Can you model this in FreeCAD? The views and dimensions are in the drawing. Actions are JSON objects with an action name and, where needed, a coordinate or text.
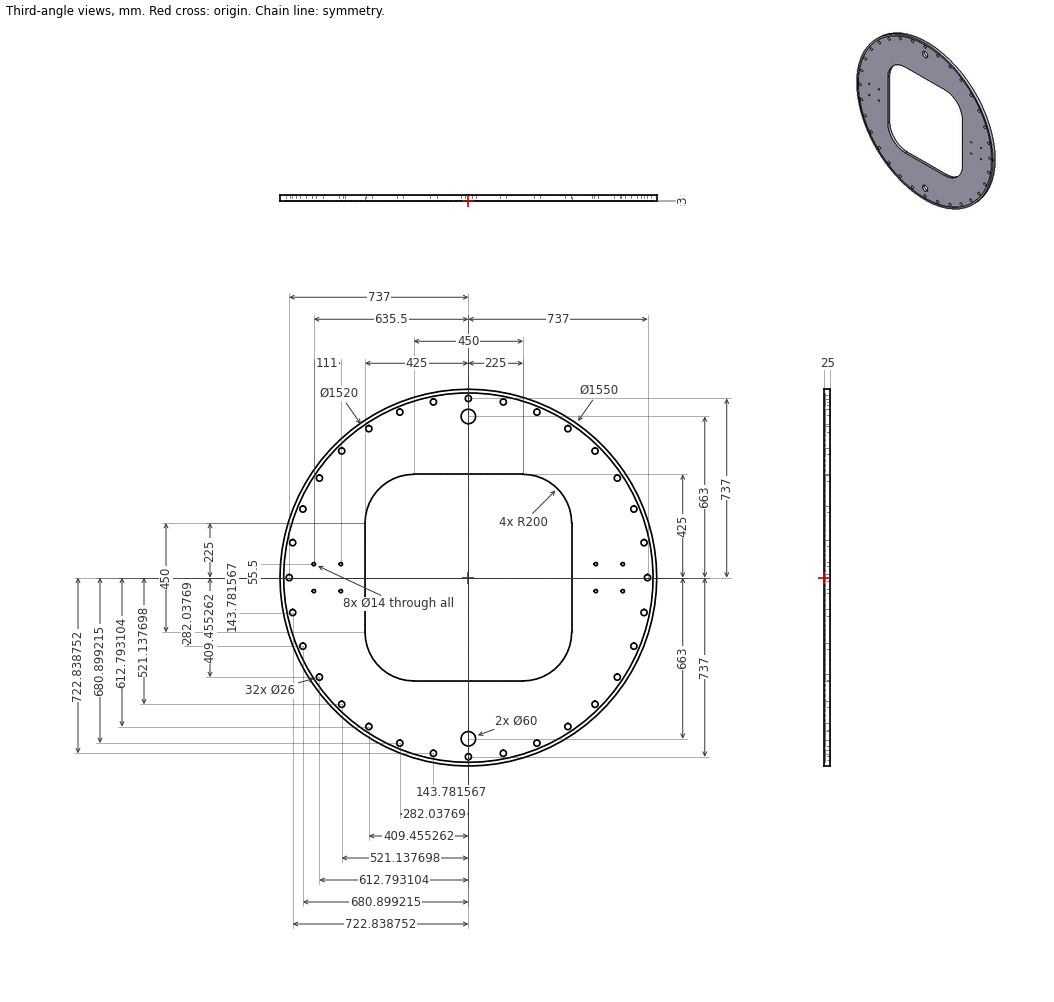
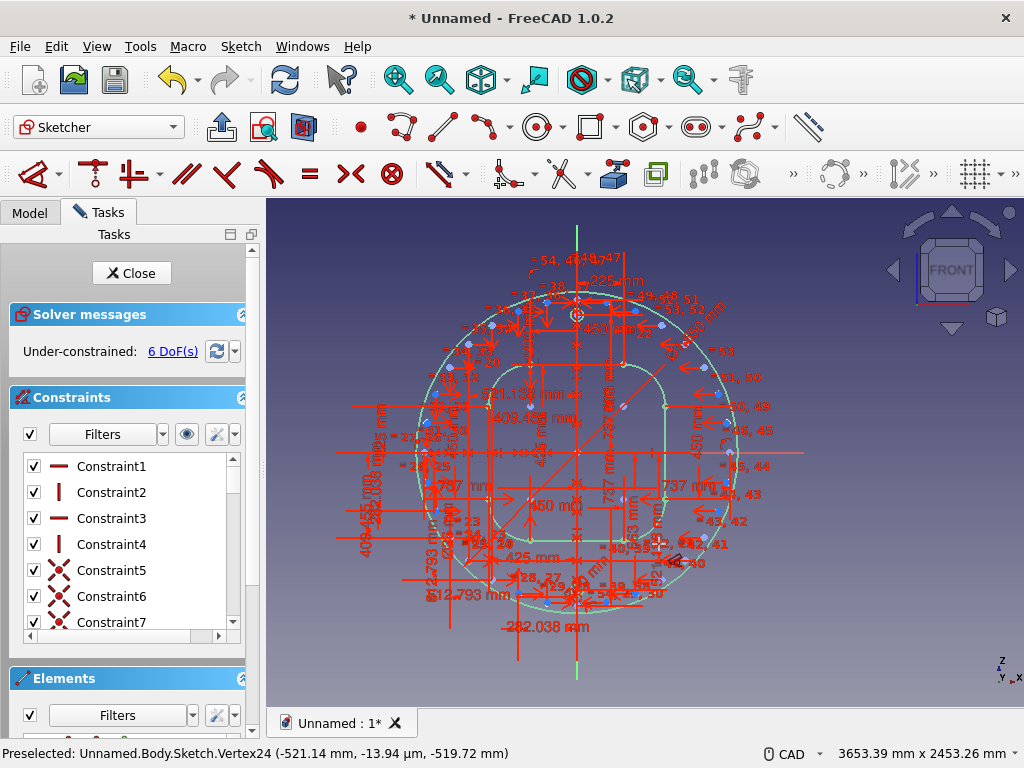
{"action": "left_click", "coordinate": [436, 511]}
{"action": "left_click", "coordinate": [474, 371]}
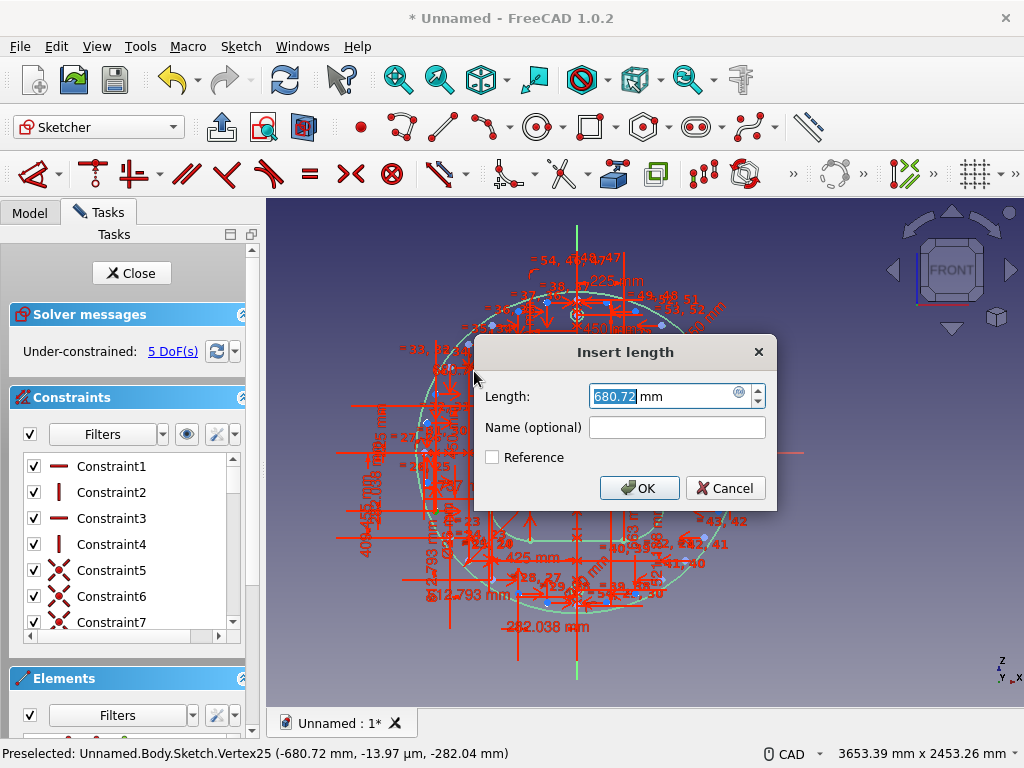
{"action": "type", "text": "680.899215"}
{"action": "key", "text": "Return"}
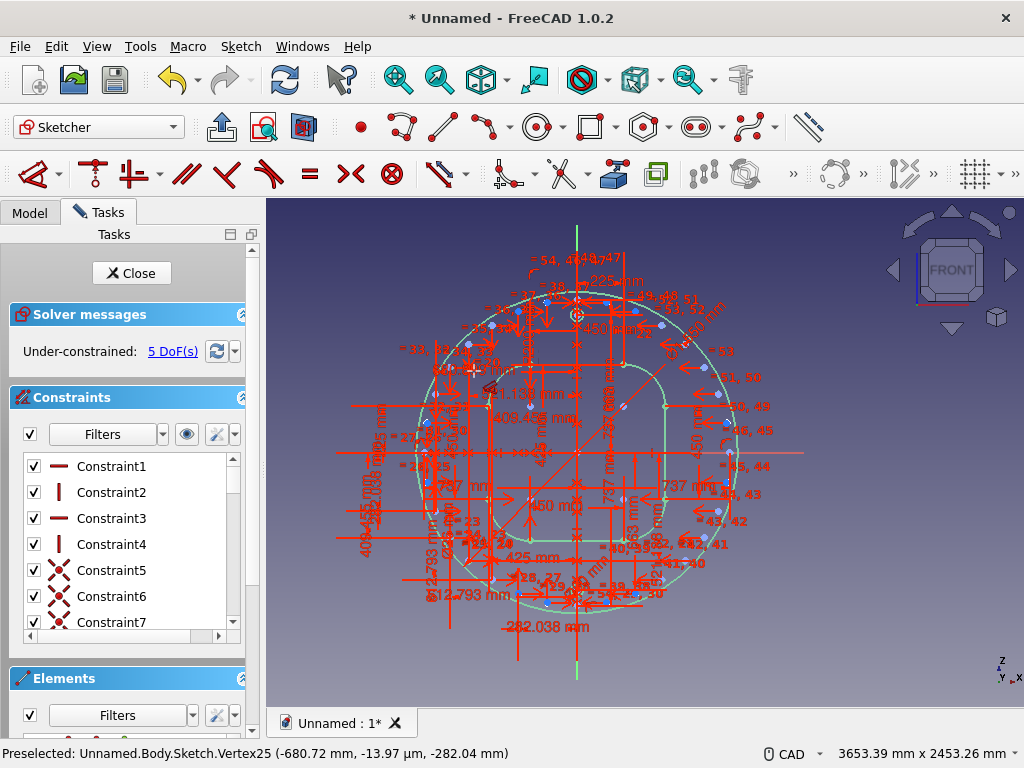
{"action": "left_click", "coordinate": [427, 483]}
{"action": "left_click", "coordinate": [450, 323]}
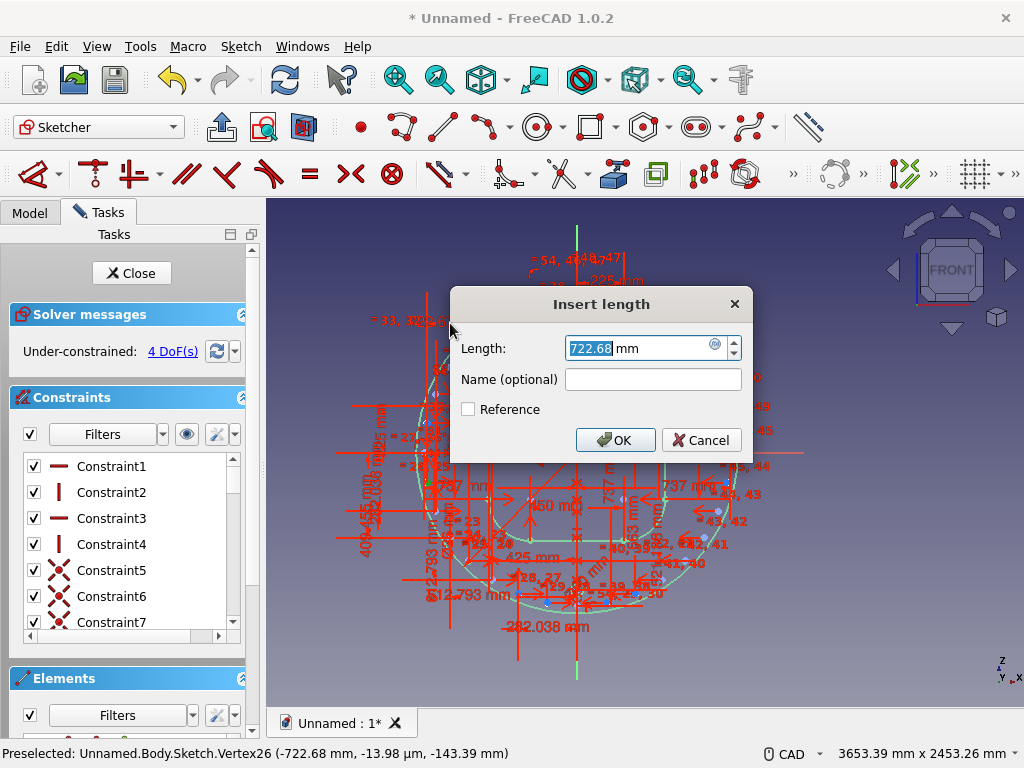
{"action": "type", "text": "722.838752"}
{"action": "key", "text": "Return"}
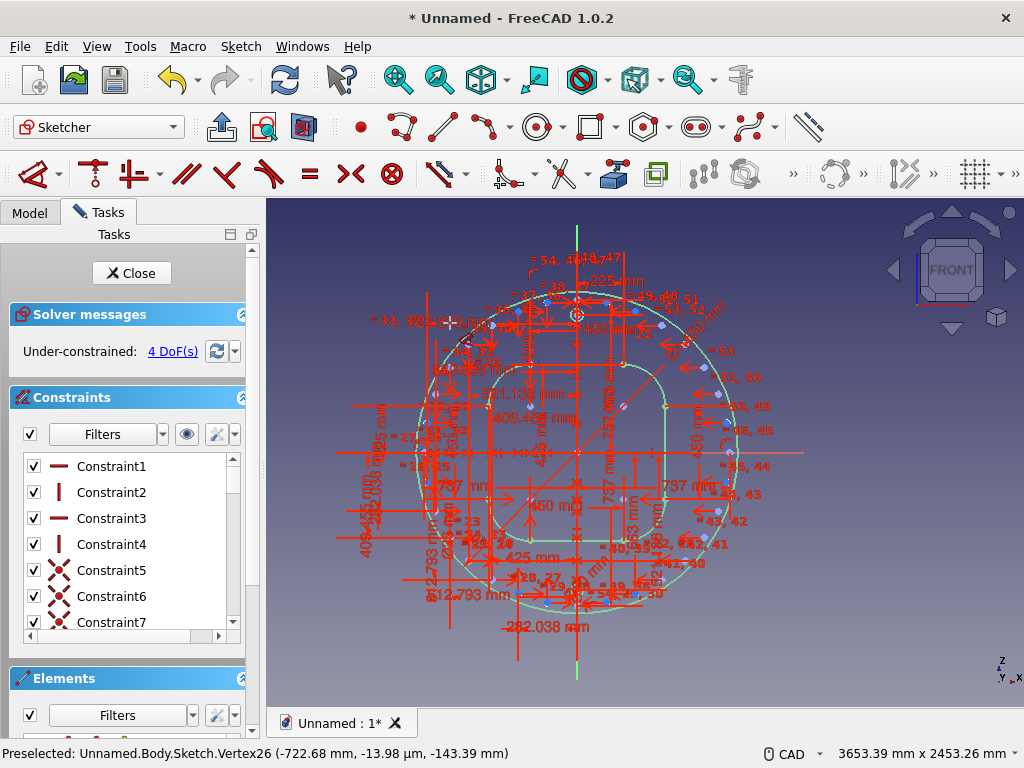
{"action": "scroll", "coordinate": [427, 483], "scroll_direction": "up", "scroll_amount": 2}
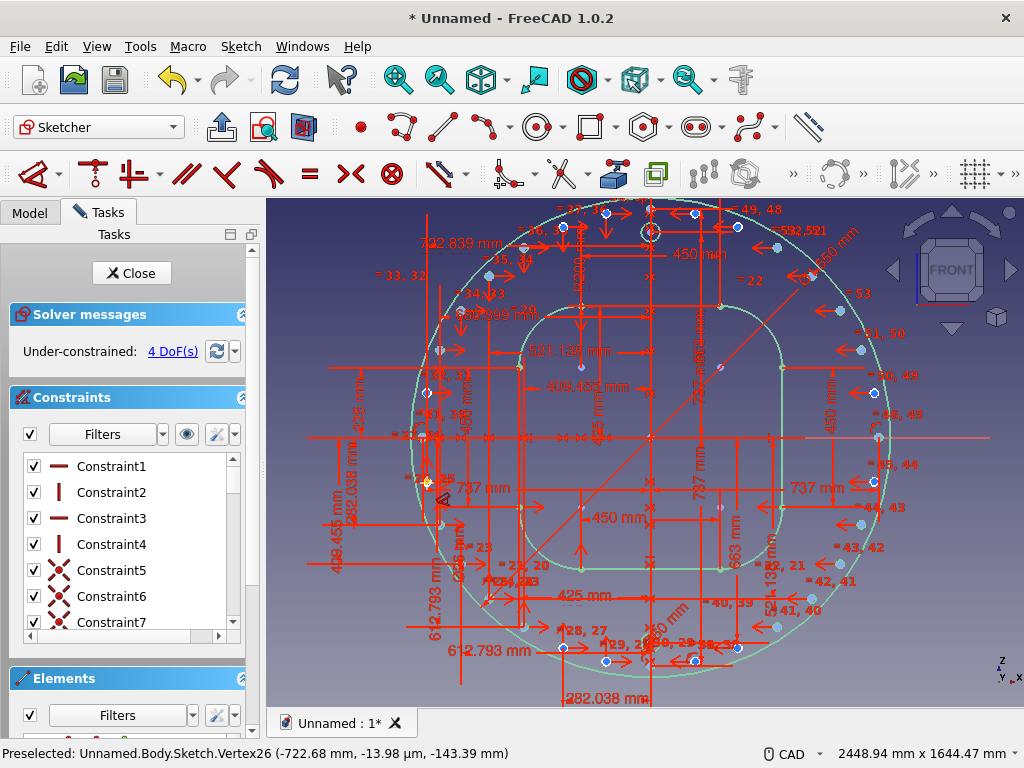
{"action": "left_click", "coordinate": [427, 482]}
{"action": "left_click", "coordinate": [393, 460]}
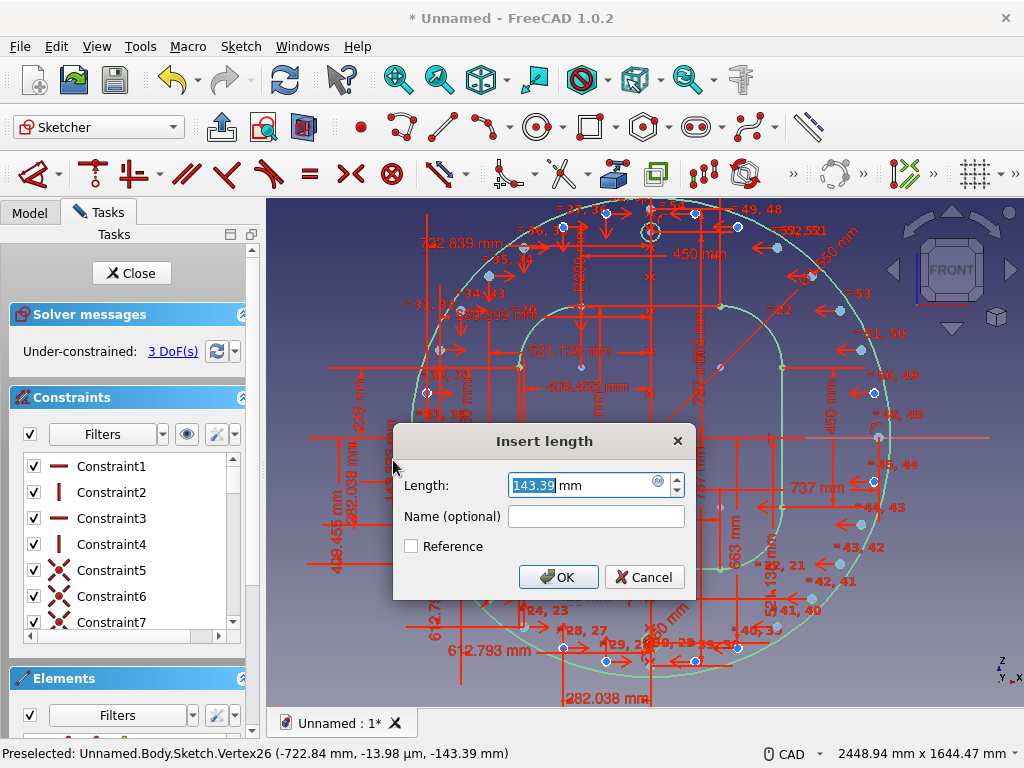
{"action": "type", "text": "143.781567"}
{"action": "key", "text": "Return"}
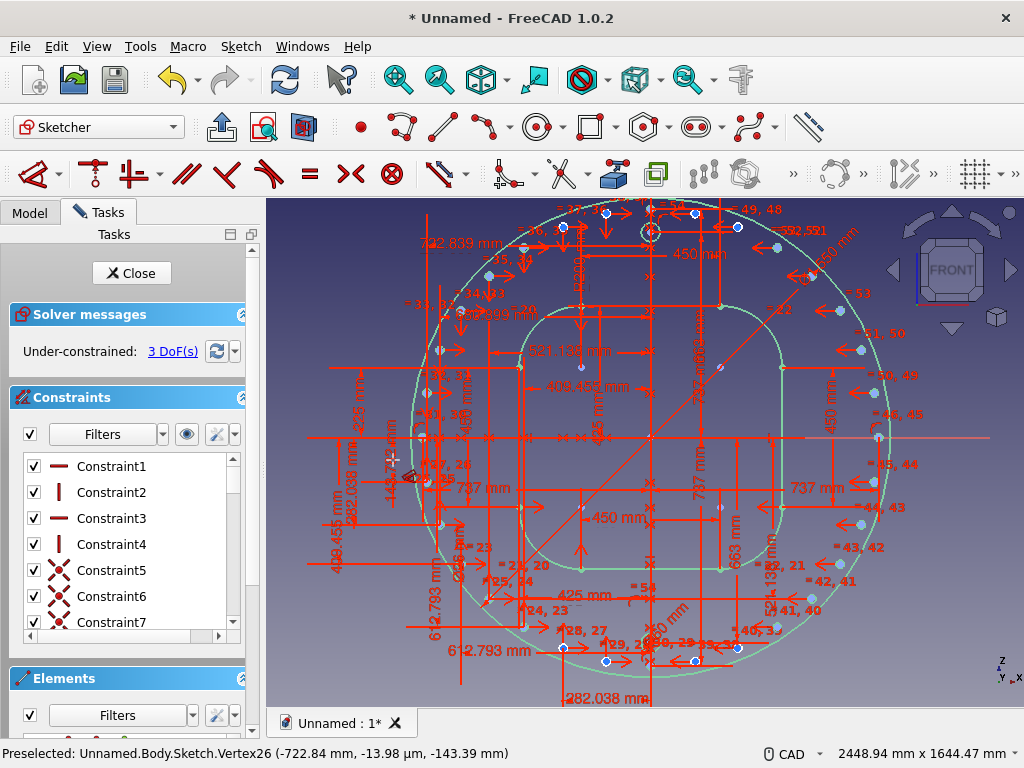
{"action": "left_click", "coordinate": [563, 648]}
{"action": "left_click", "coordinate": [685, 494]}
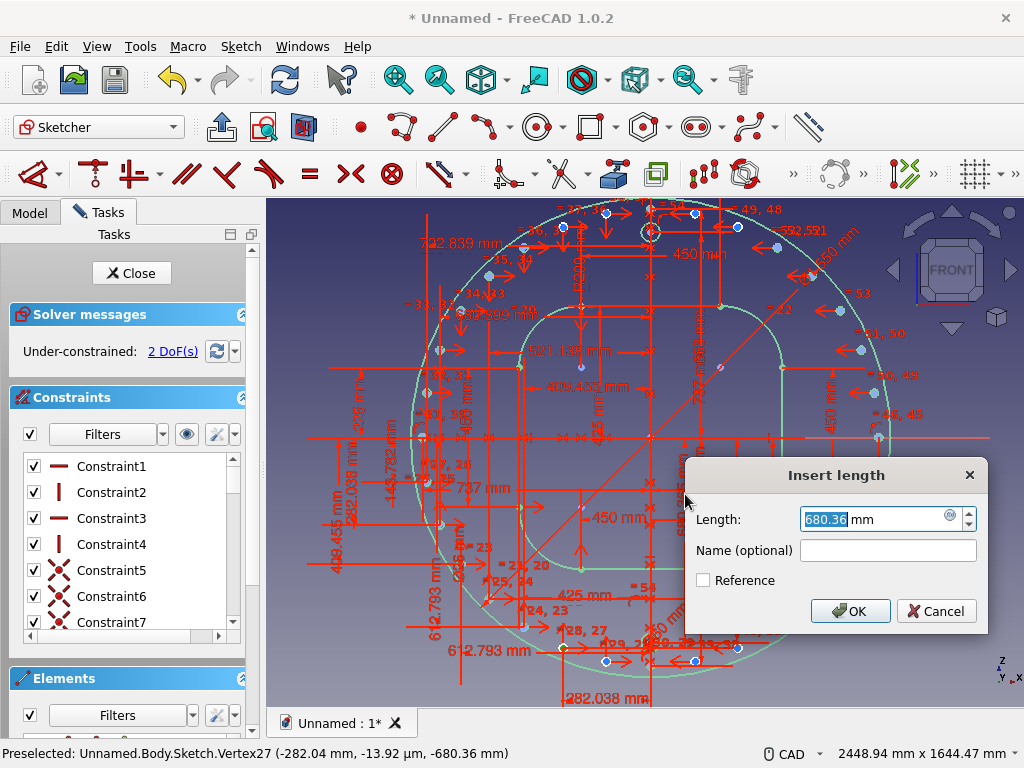
{"action": "type", "text": "680.899215"}
{"action": "key", "text": "Return"}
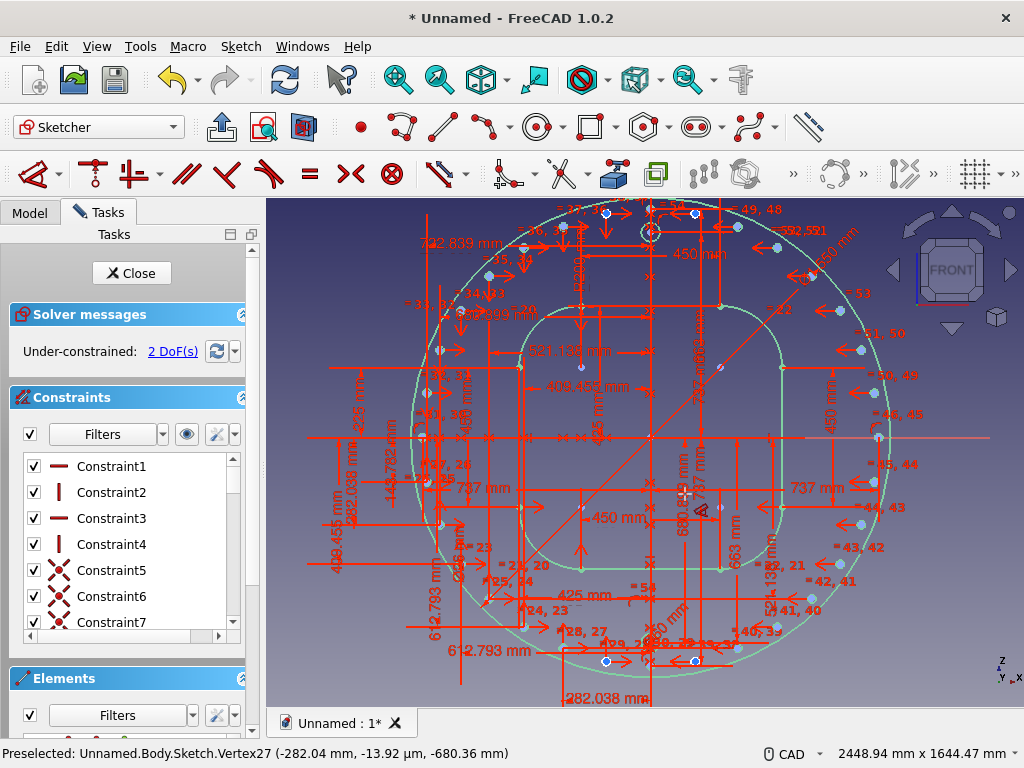
{"action": "left_click", "coordinate": [606, 662]}
{"action": "left_click", "coordinate": [628, 284]}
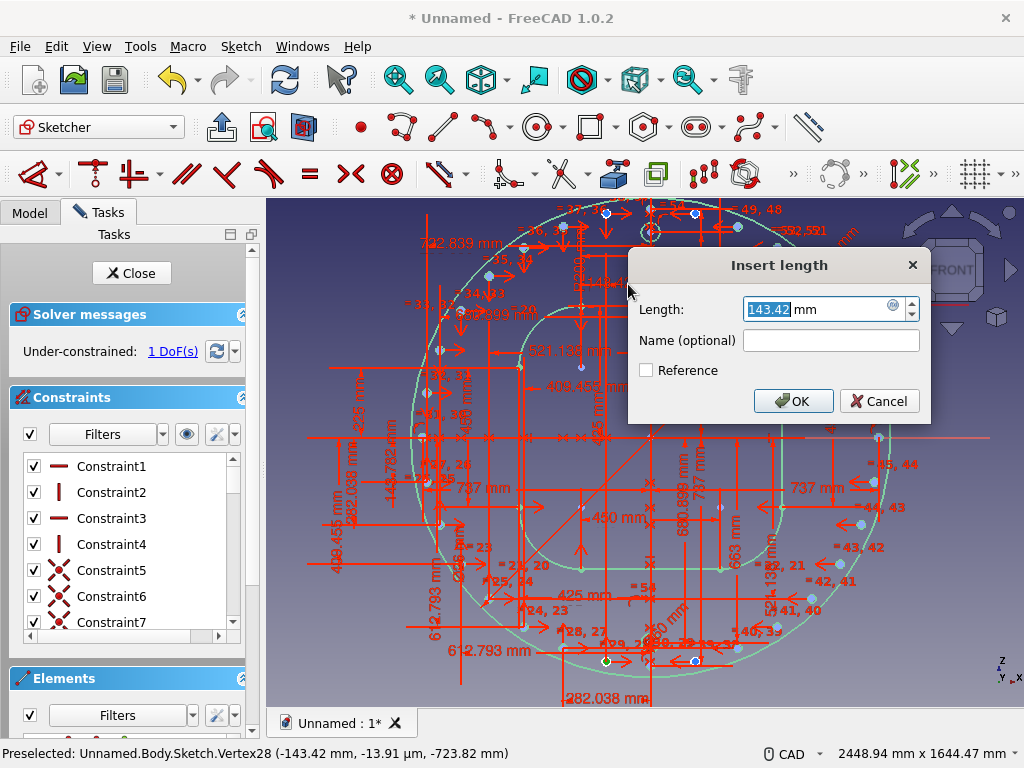
{"action": "type", "text": "143.781567"}
{"action": "key", "text": "Return"}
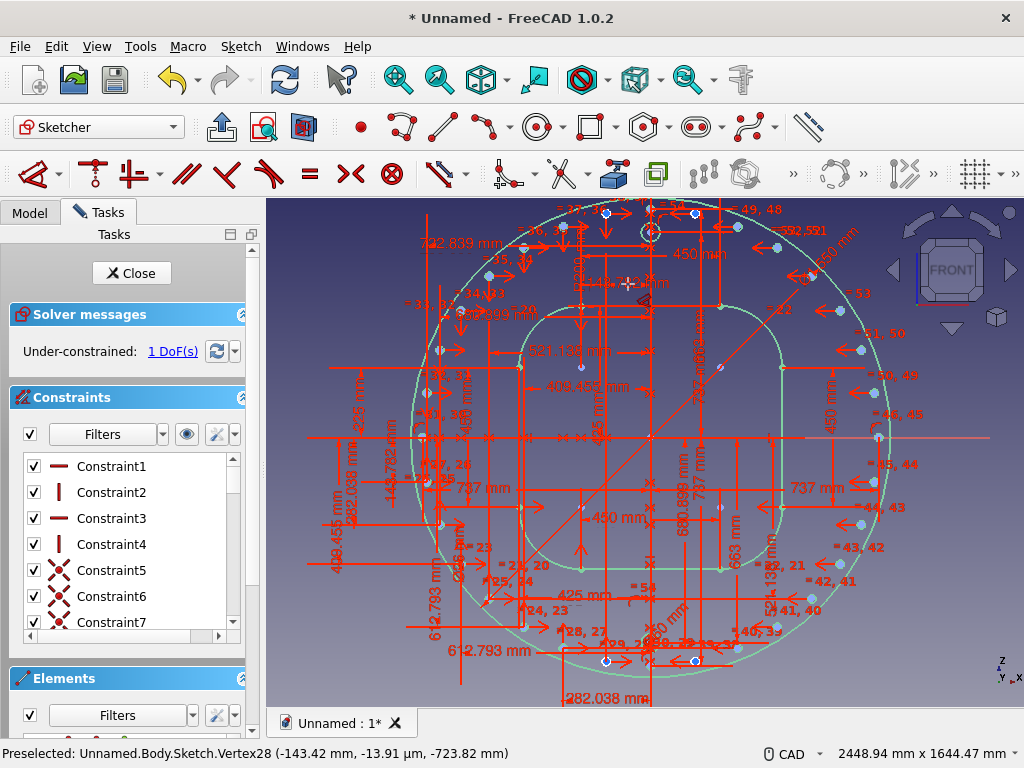
{"action": "left_click", "coordinate": [606, 662]}
{"action": "left_click", "coordinate": [572, 550]}